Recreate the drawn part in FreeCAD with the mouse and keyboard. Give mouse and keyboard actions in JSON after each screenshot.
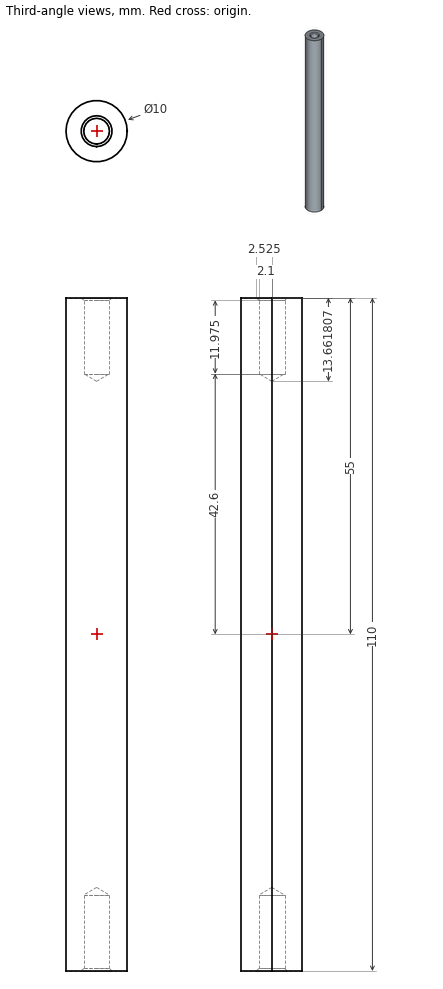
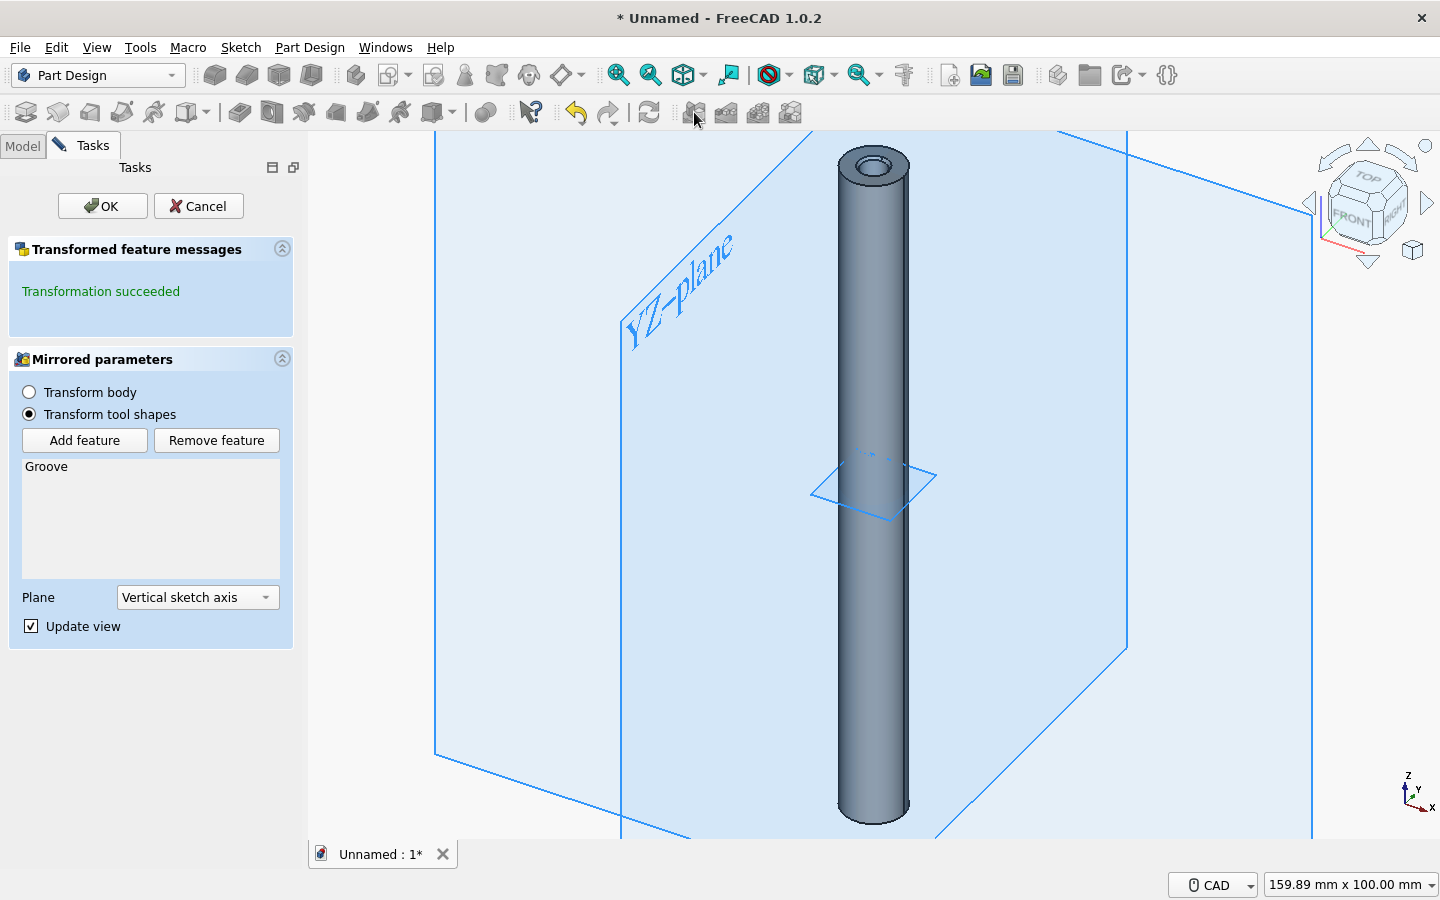
{"action": "left_click", "coordinate": [198, 598]}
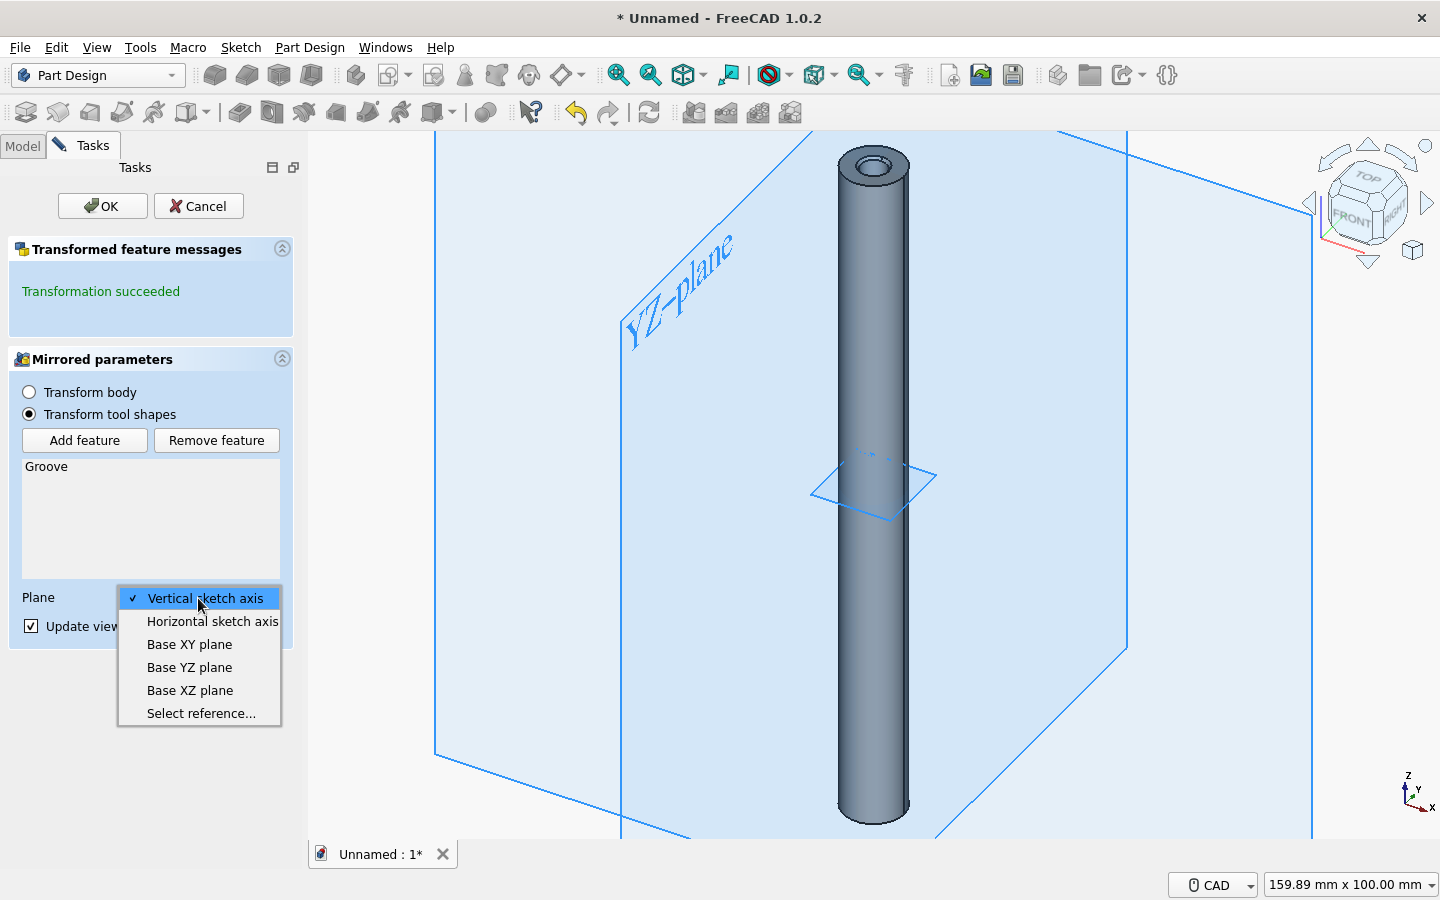
{"action": "left_click", "coordinate": [198, 644]}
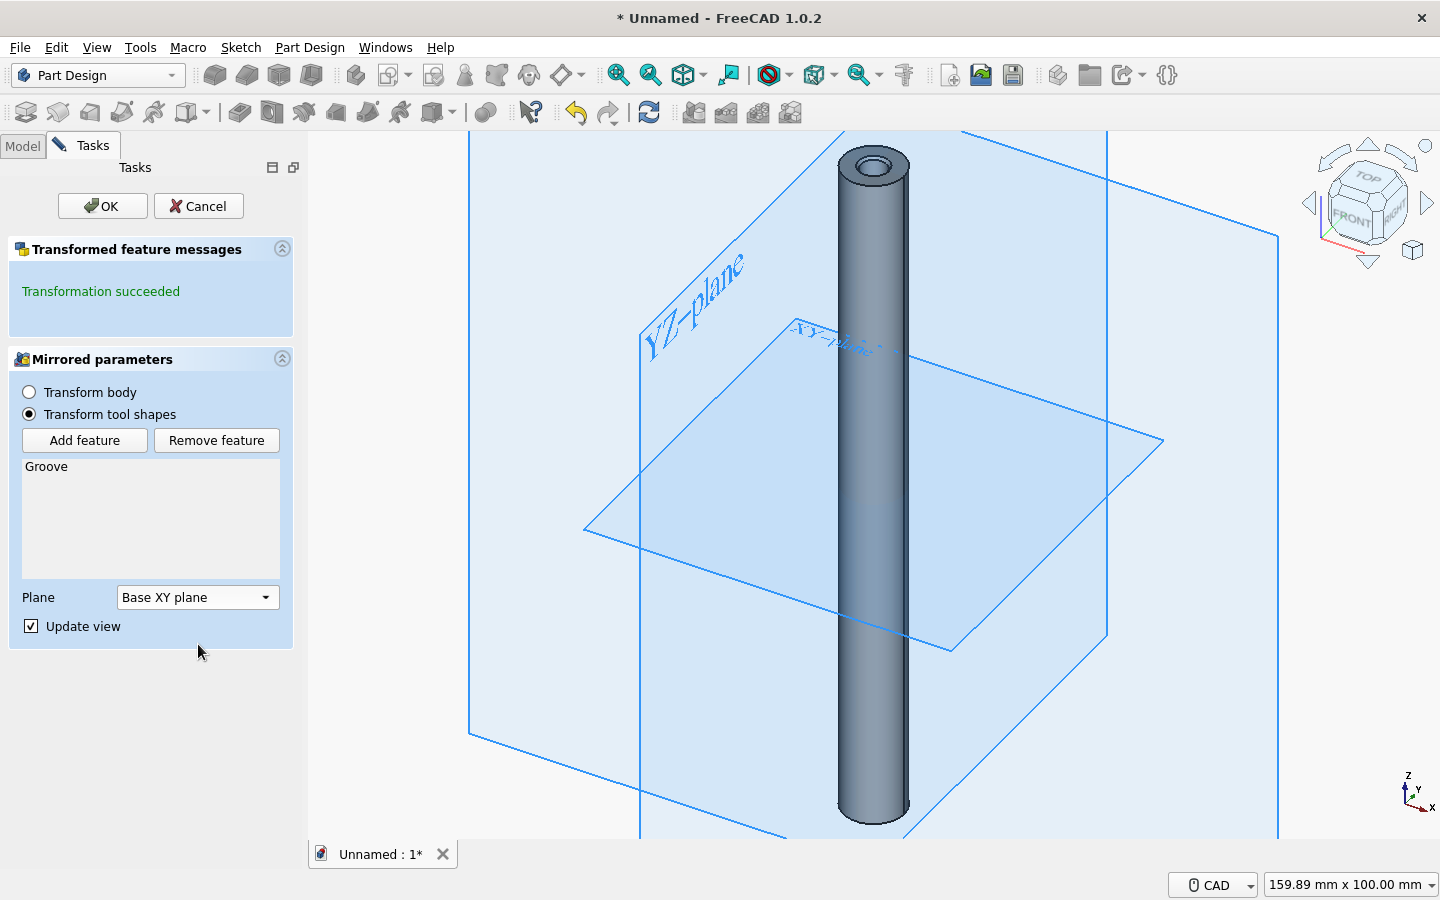
{"action": "left_click", "coordinate": [103, 206]}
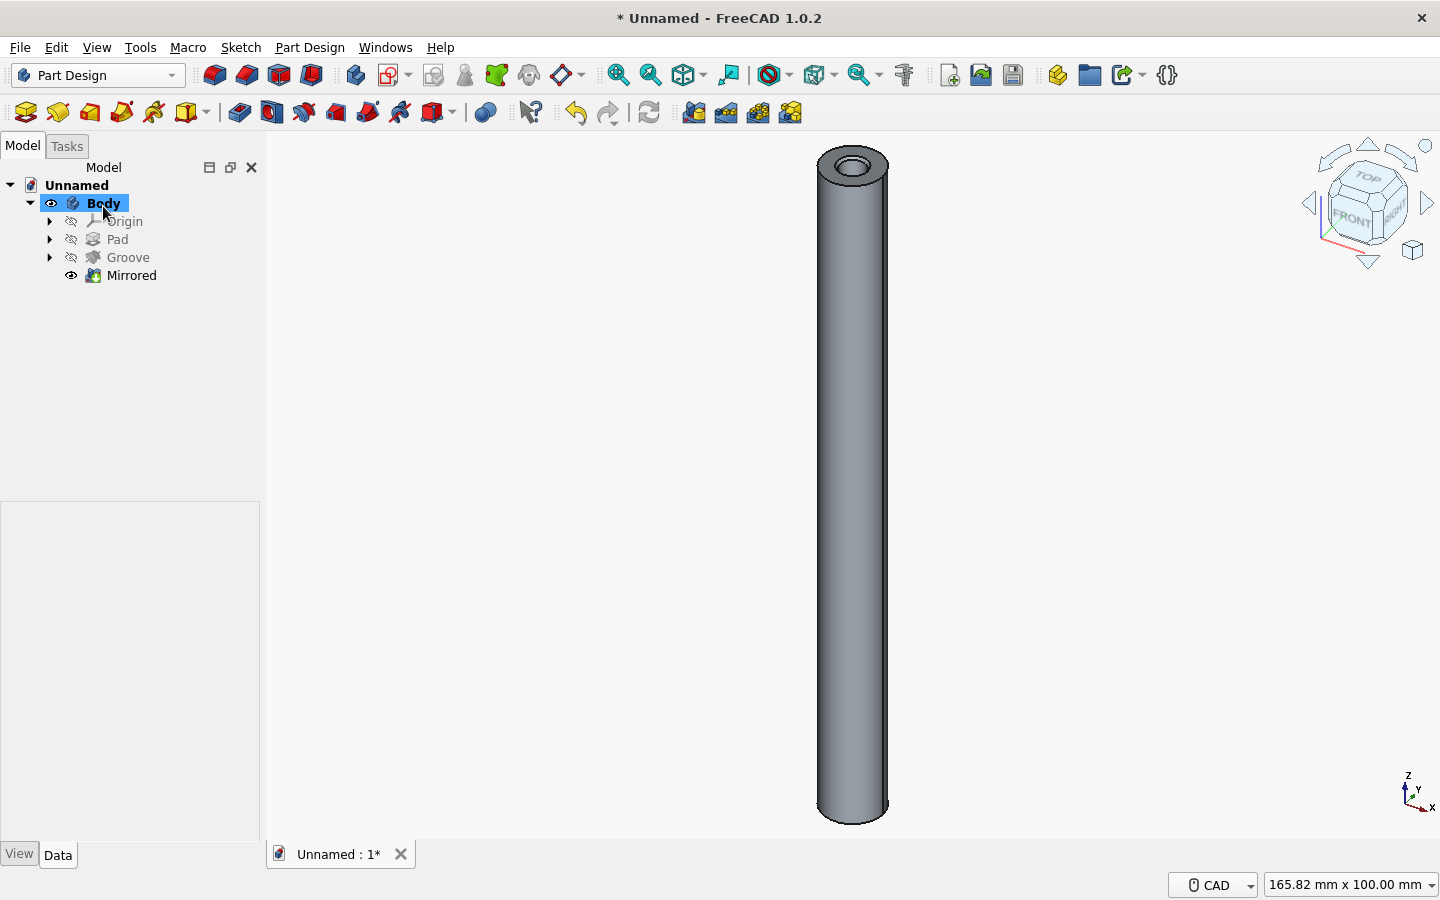
{"action": "key", "text": "0"}